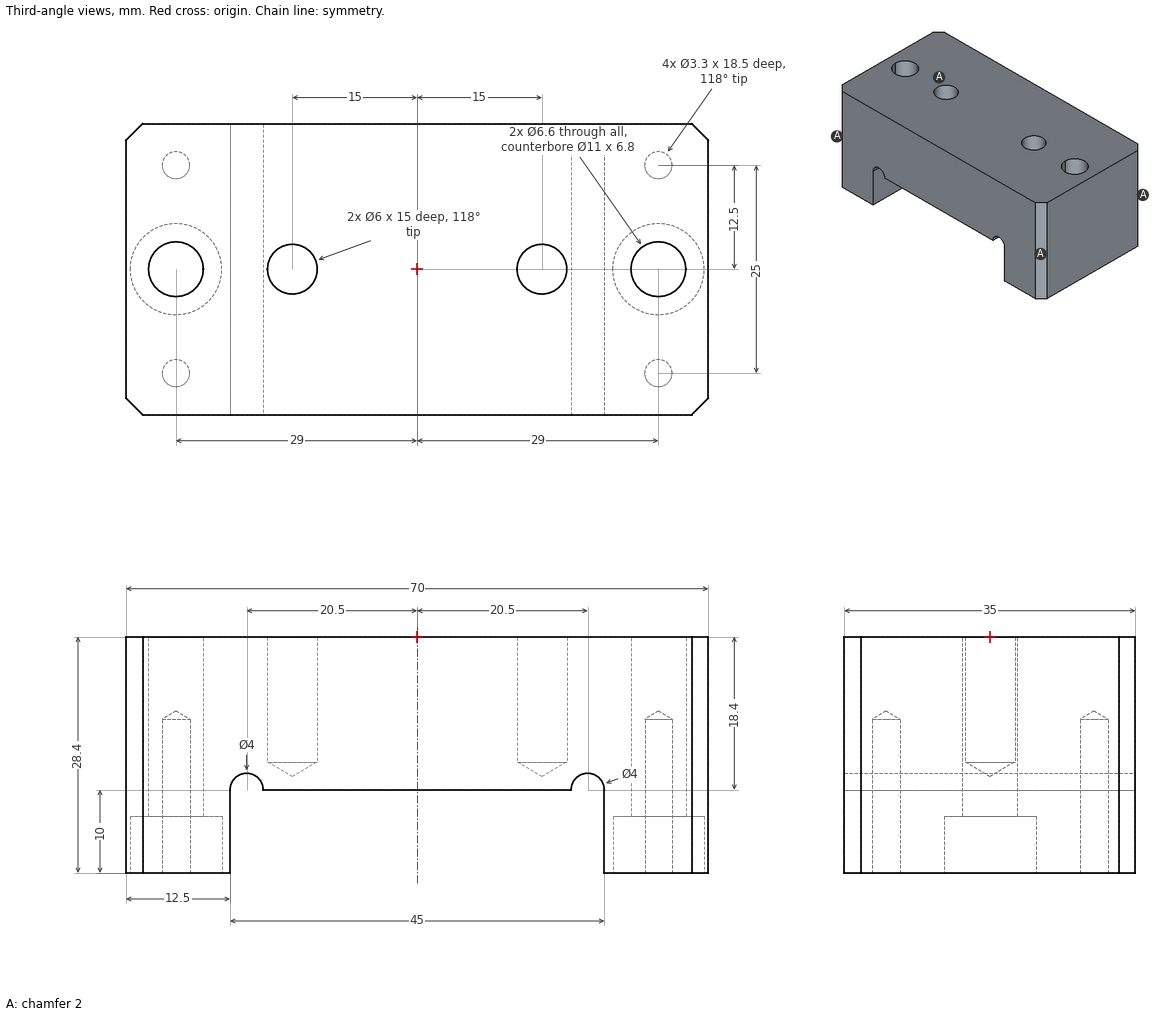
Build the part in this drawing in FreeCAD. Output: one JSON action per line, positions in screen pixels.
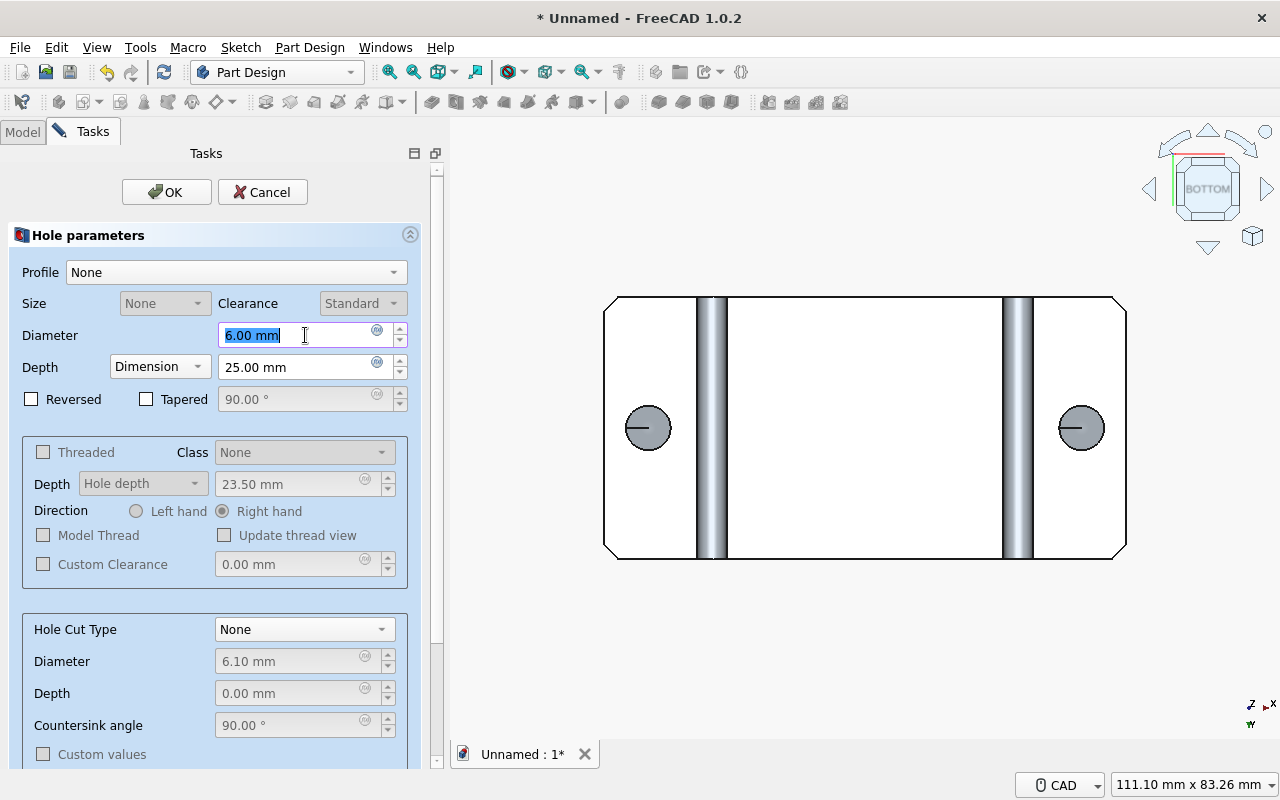
{"action": "type", "text": "6.6"}
{"action": "key", "text": "Tab"}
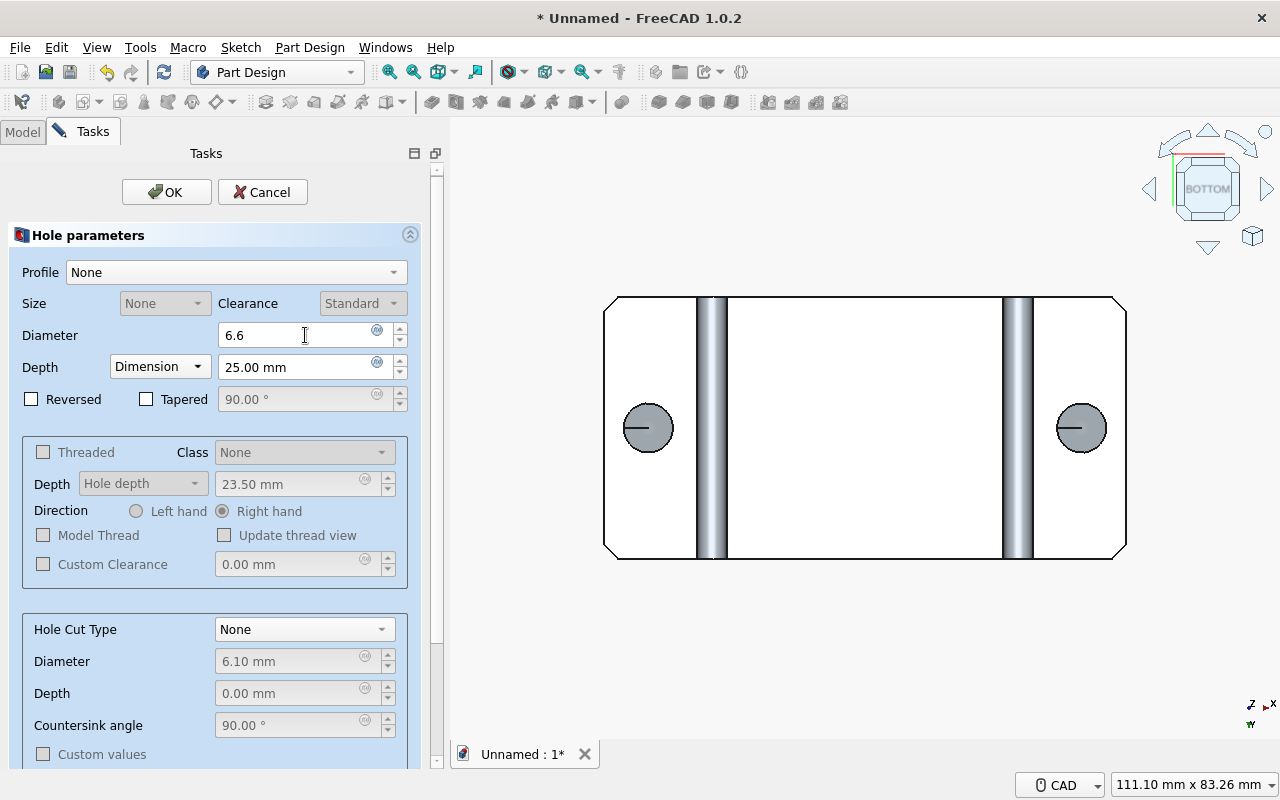
{"action": "left_click", "coordinate": [161, 366]}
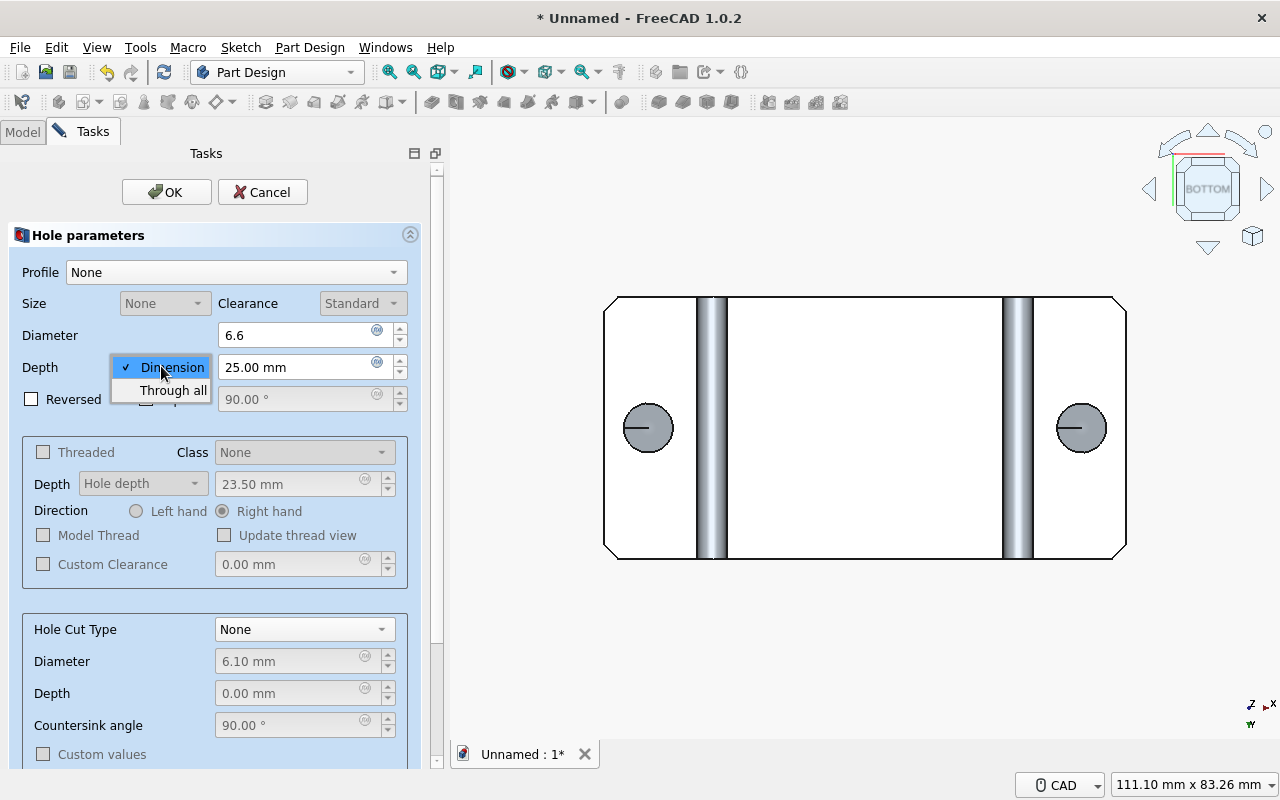
{"action": "left_click", "coordinate": [160, 390]}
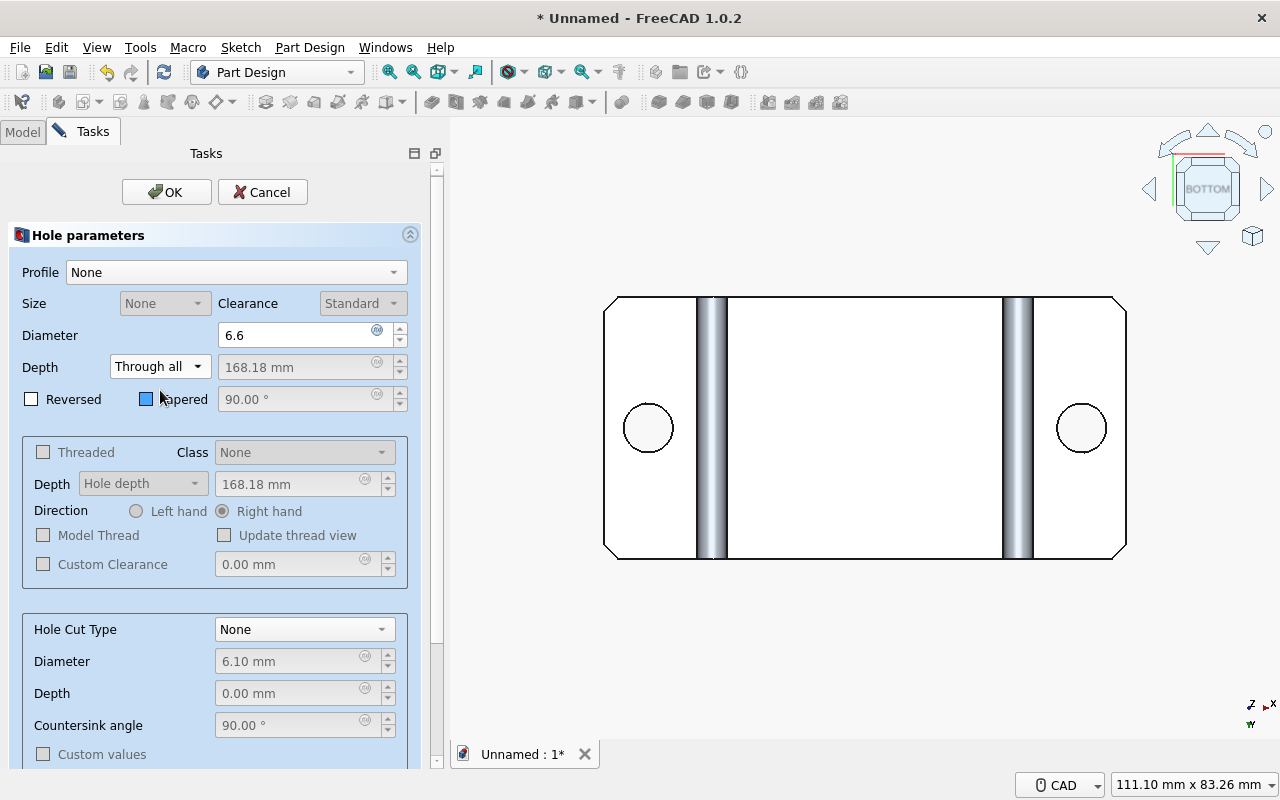
{"action": "left_click", "coordinate": [306, 630]}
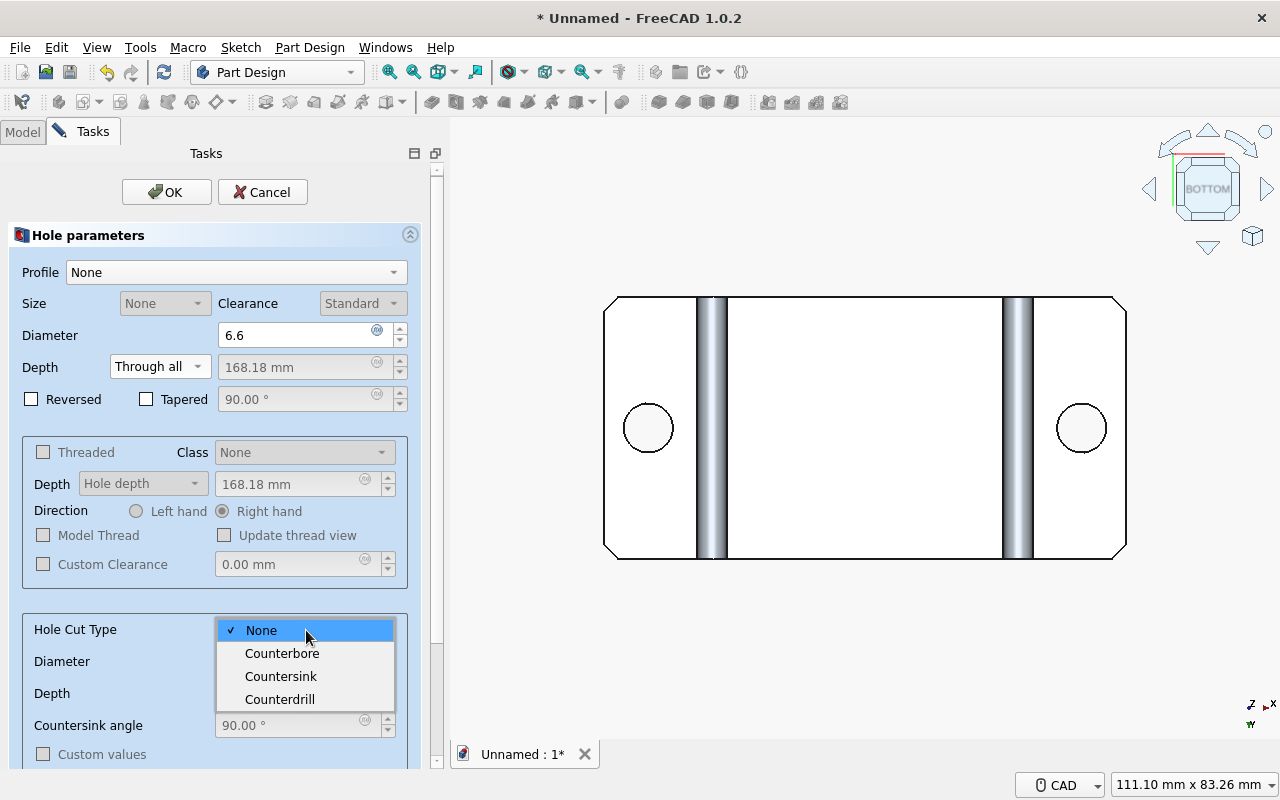
{"action": "left_click", "coordinate": [304, 654]}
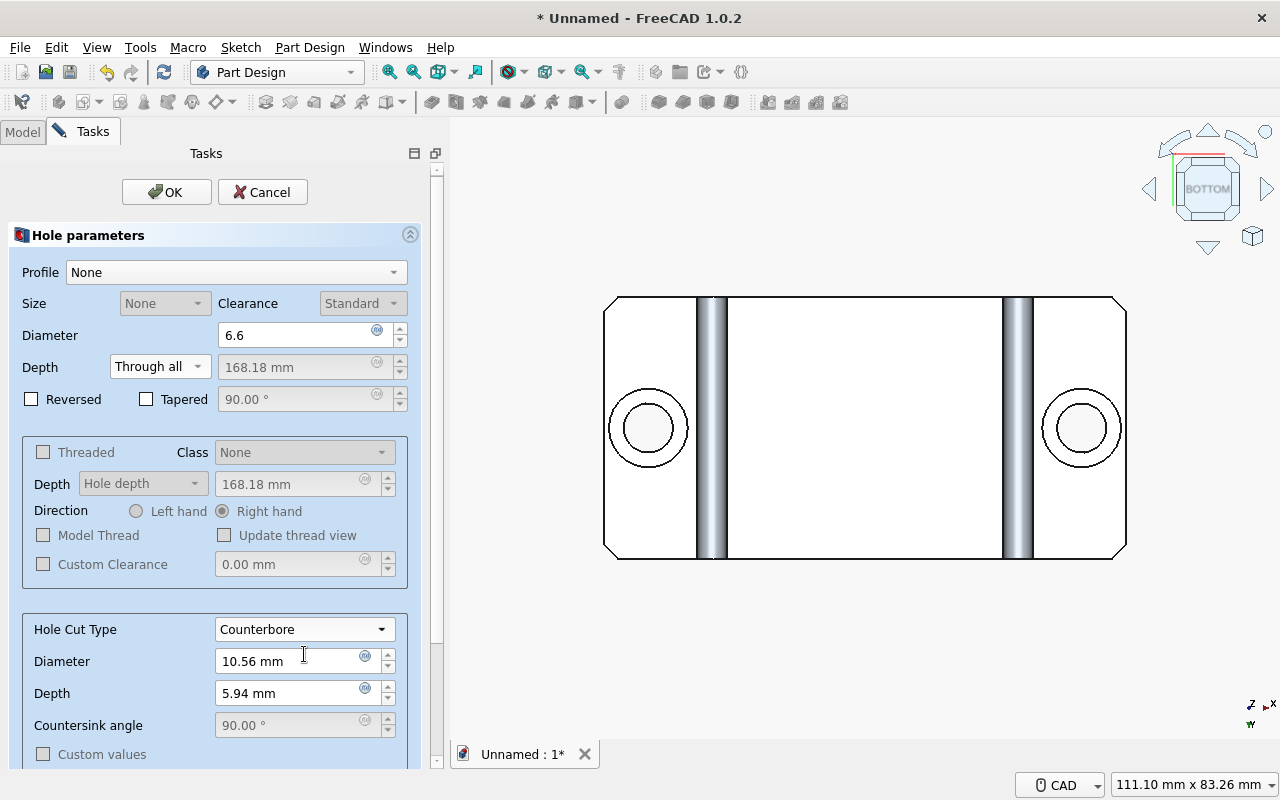
{"action": "triple_click", "coordinate": [298, 661]}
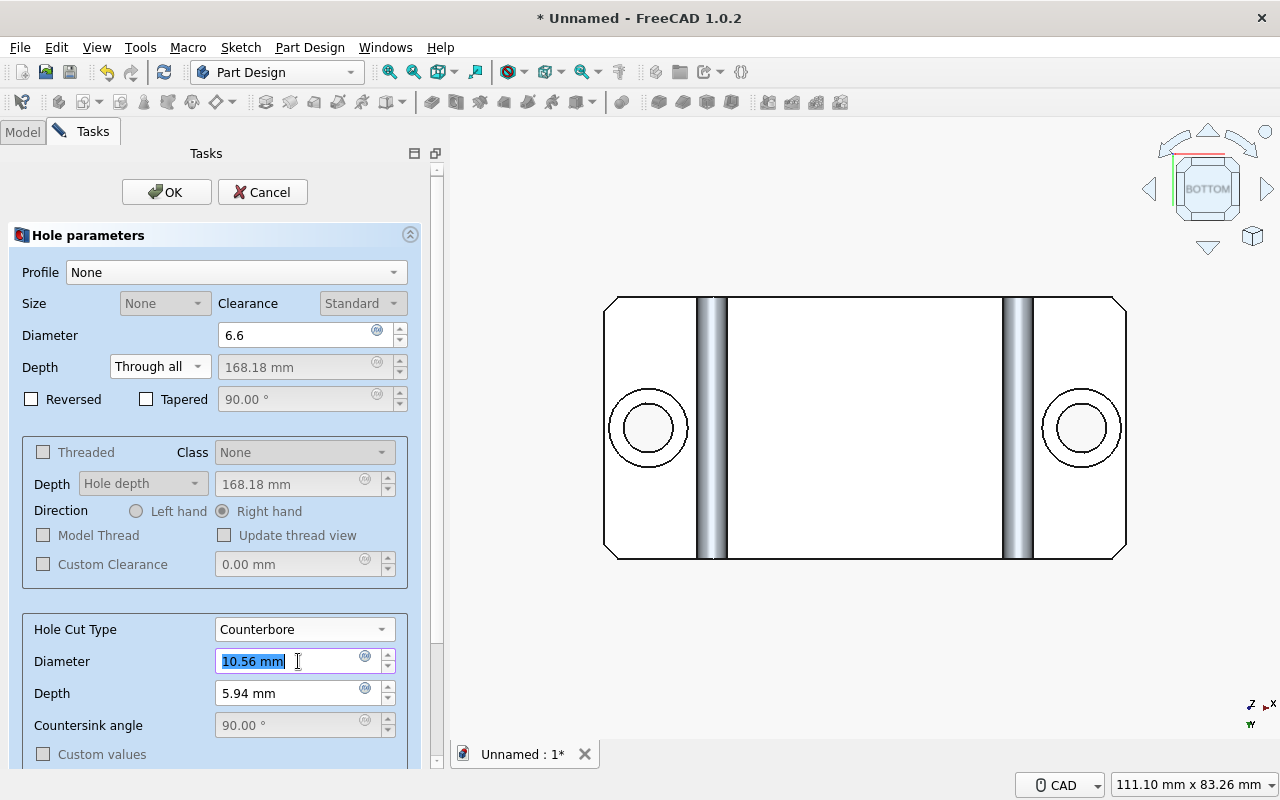
{"action": "type", "text": "11"}
{"action": "key", "text": "Tab"}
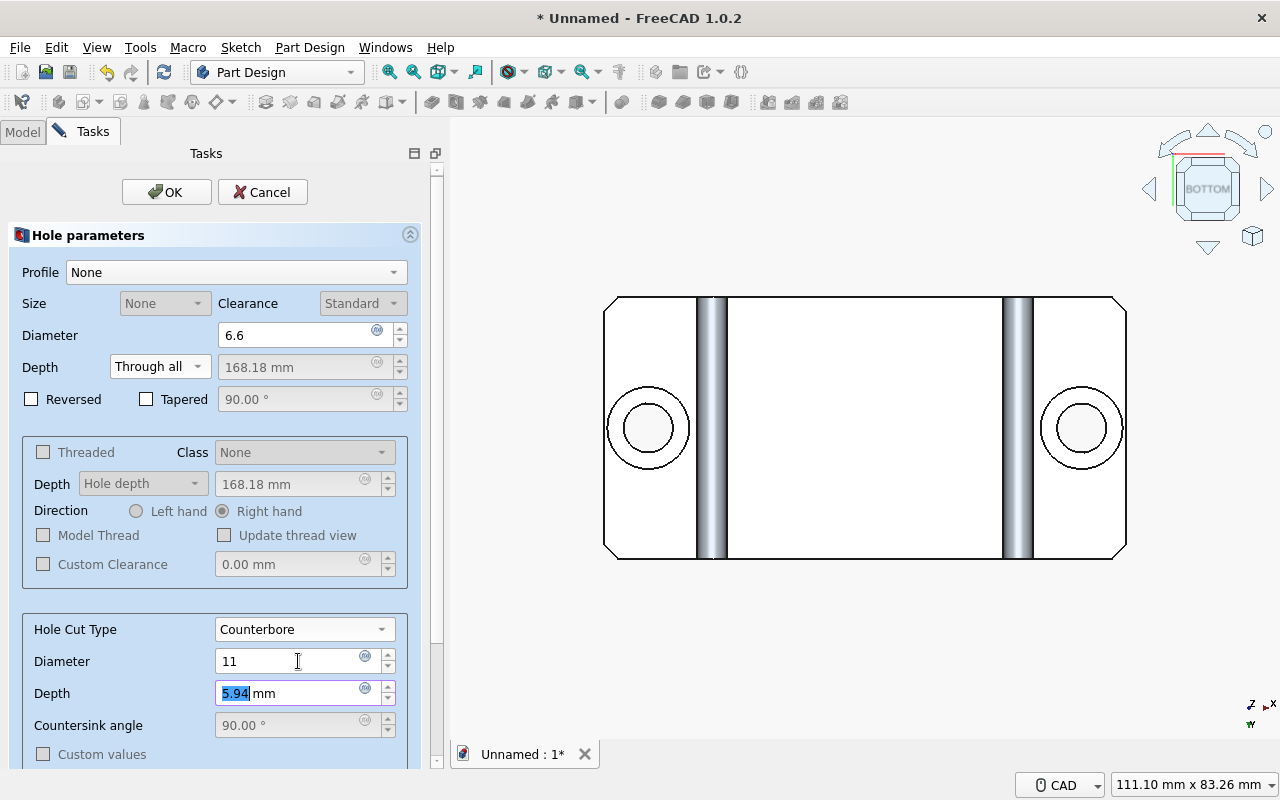
{"action": "type", "text": "6.8"}
{"action": "key", "text": "Tab"}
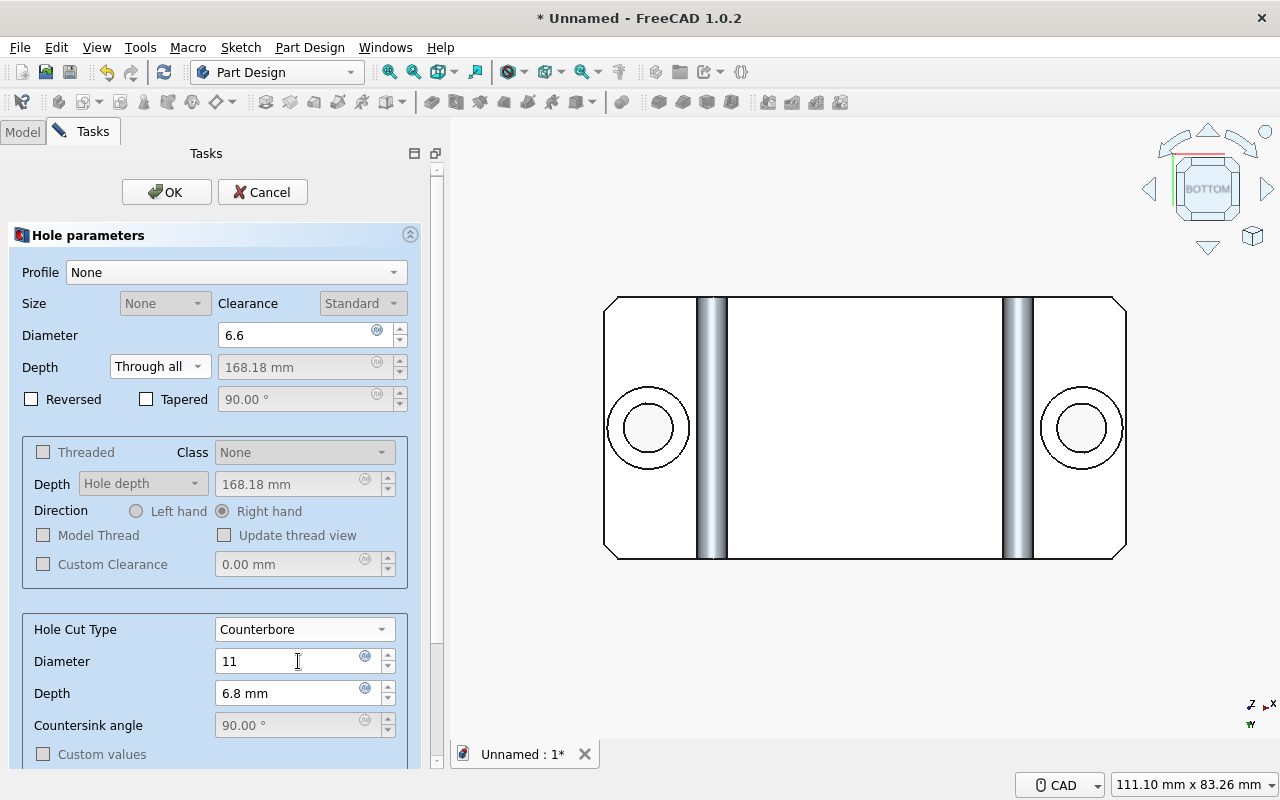
{"action": "left_click", "coordinate": [167, 192]}